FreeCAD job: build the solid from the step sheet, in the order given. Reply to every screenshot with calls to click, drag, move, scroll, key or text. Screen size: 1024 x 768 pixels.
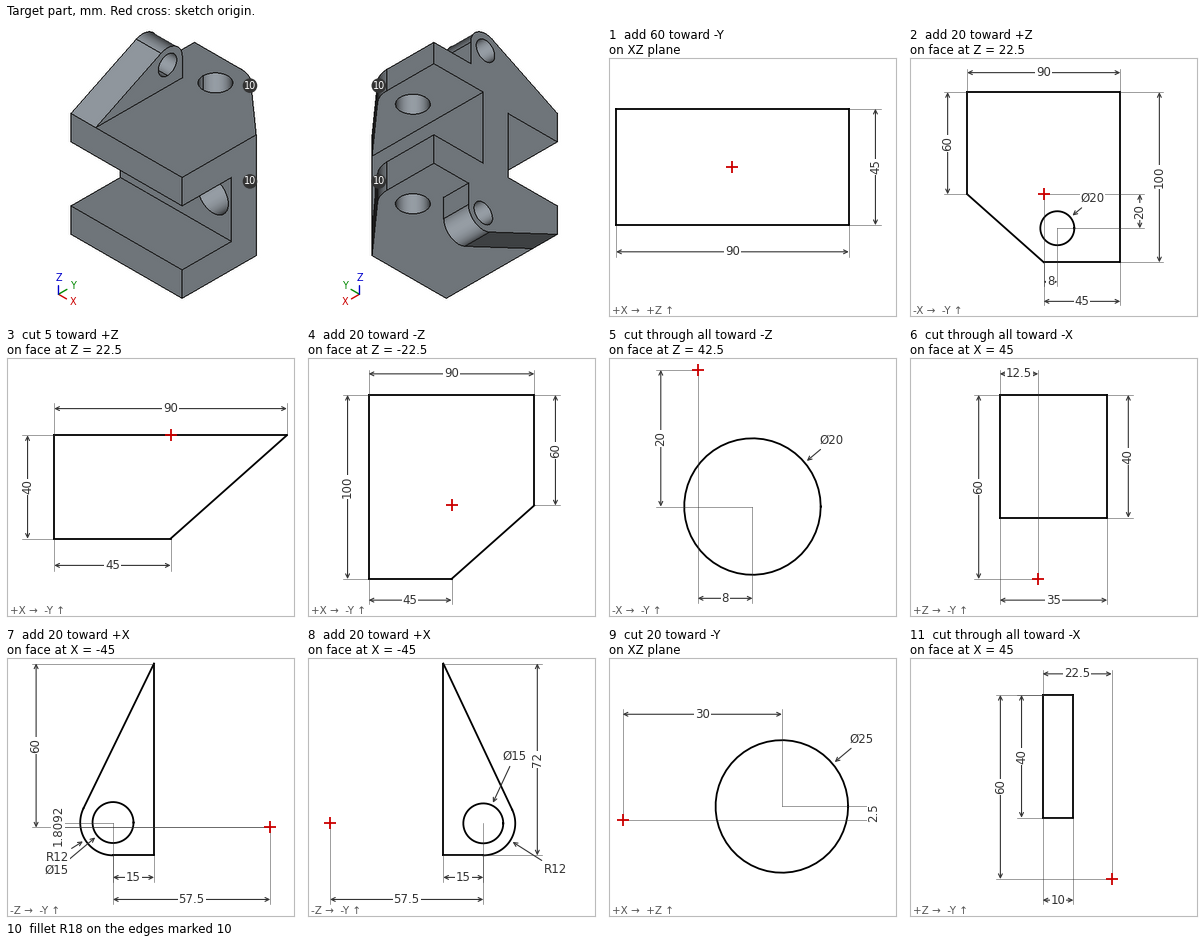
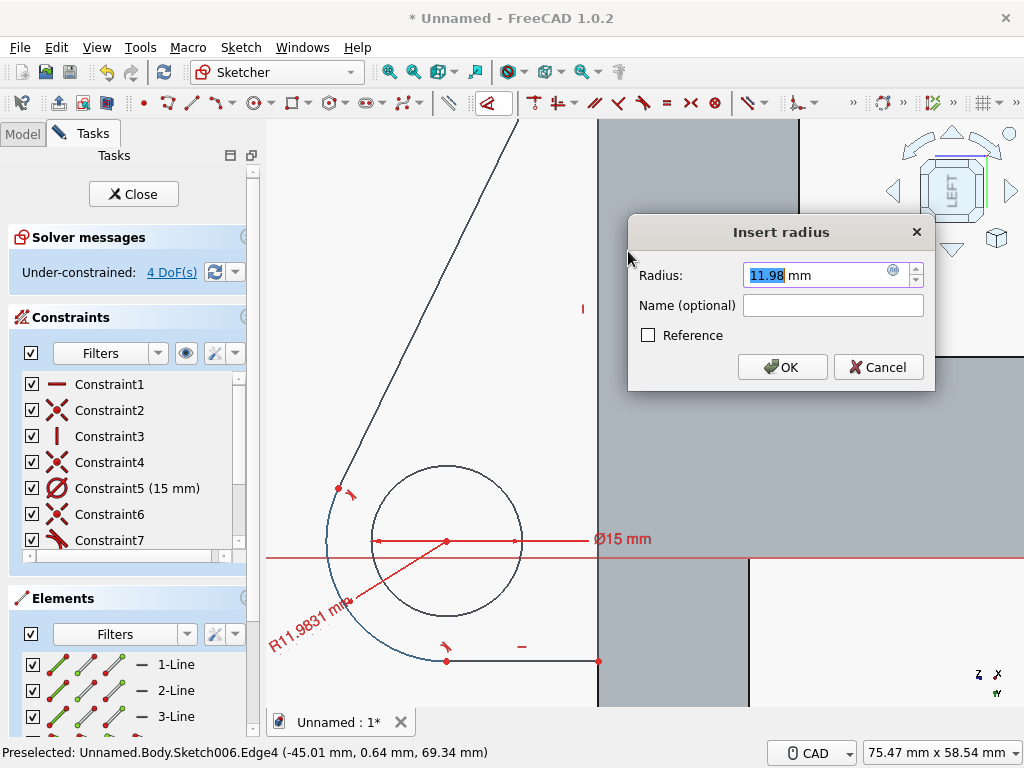
text(12)
key(Return)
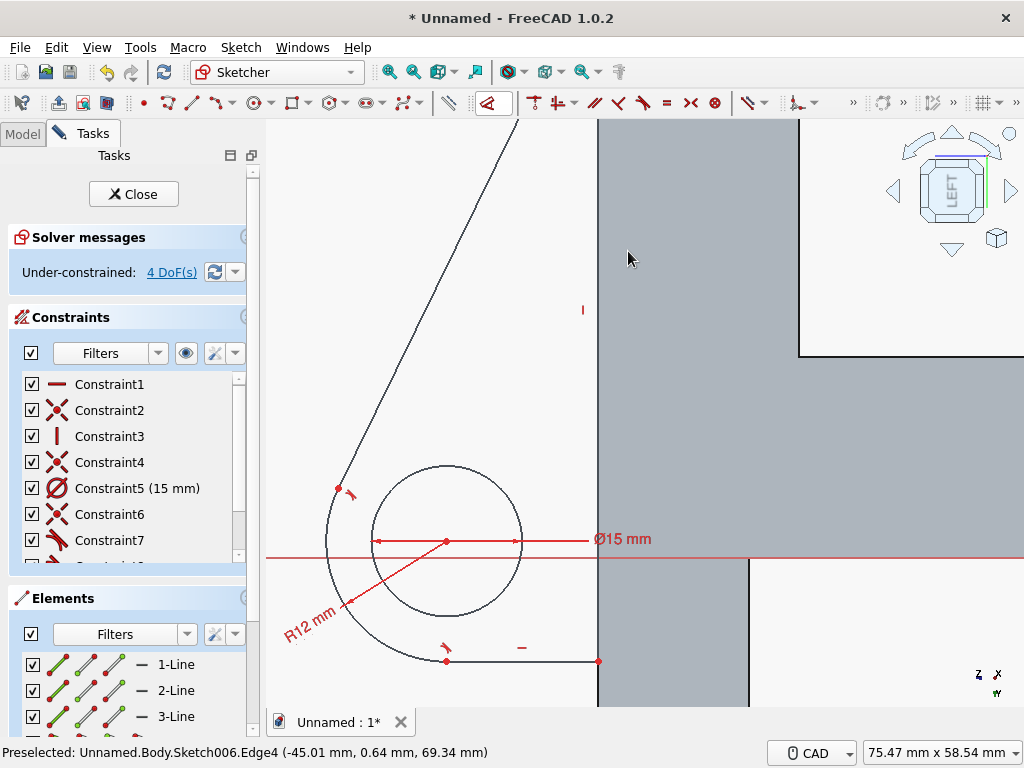
click(492, 662)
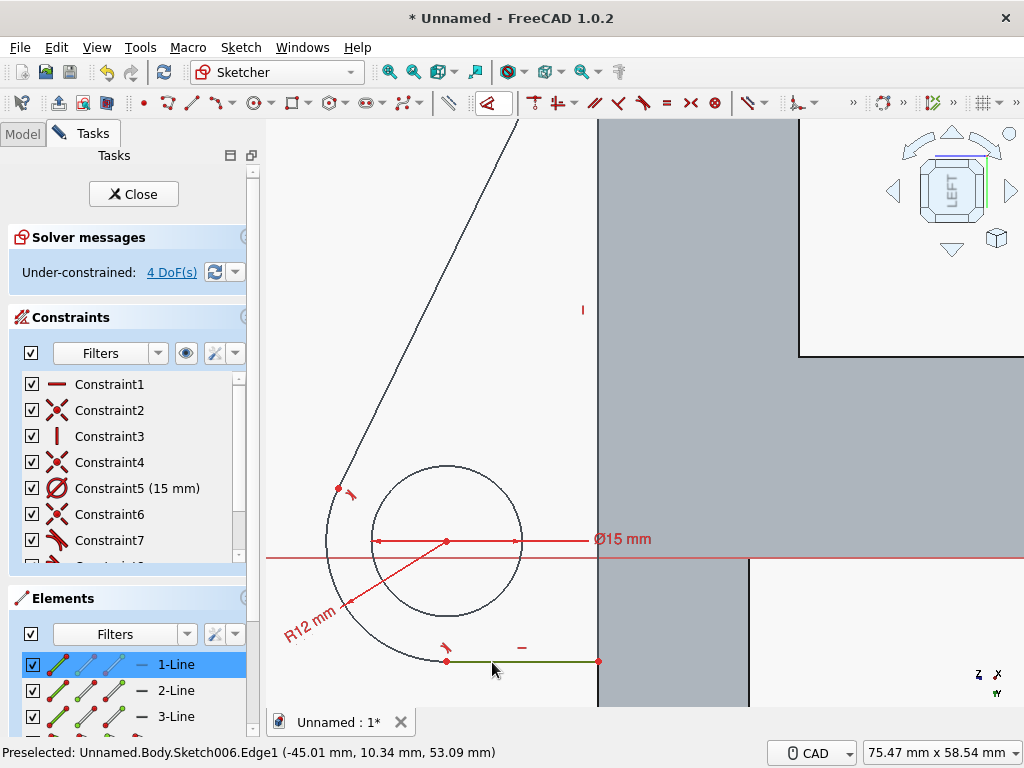
key(l)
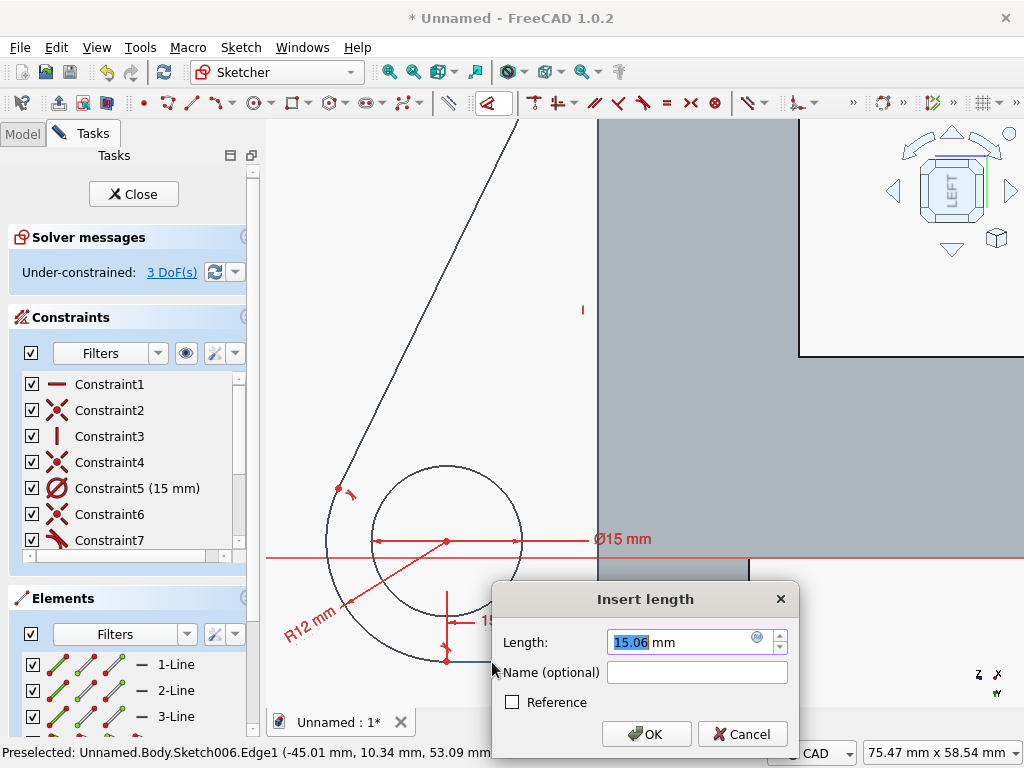
text(15)
key(Return)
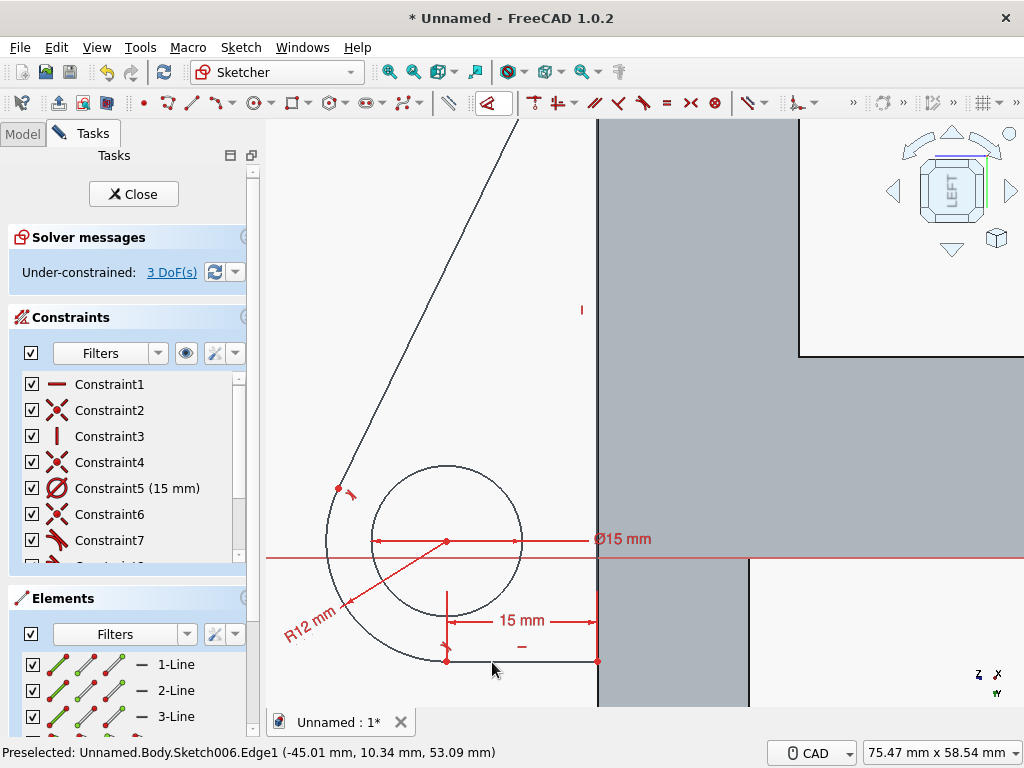
scroll(448, 541, down, 3)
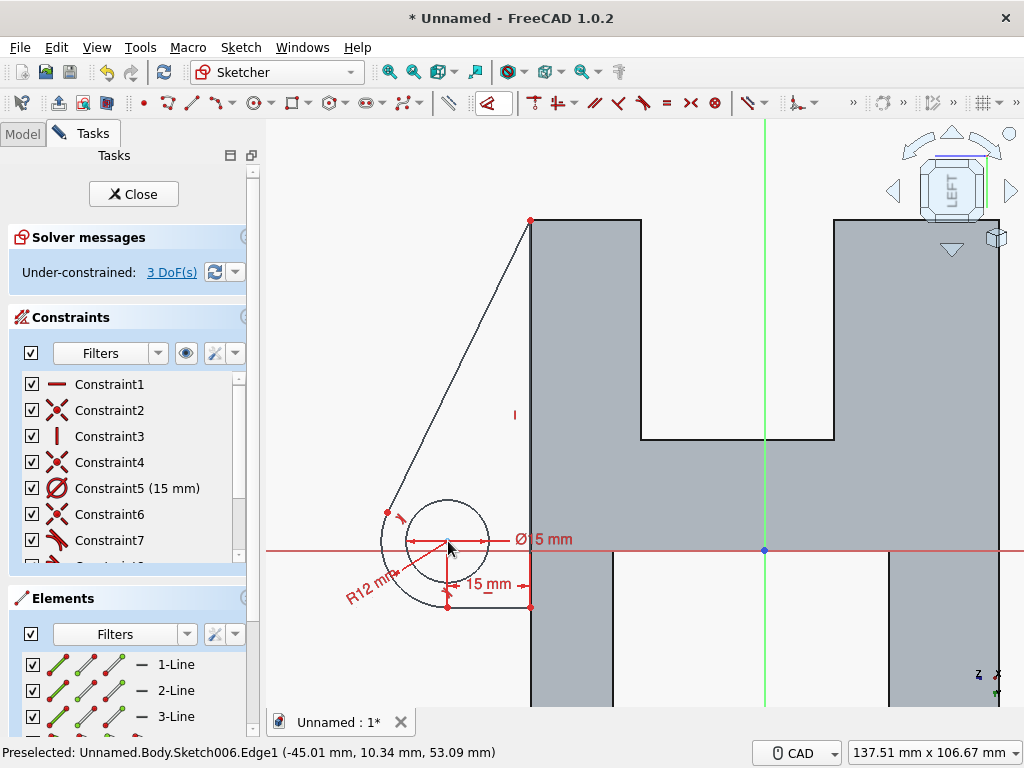
click(530, 220)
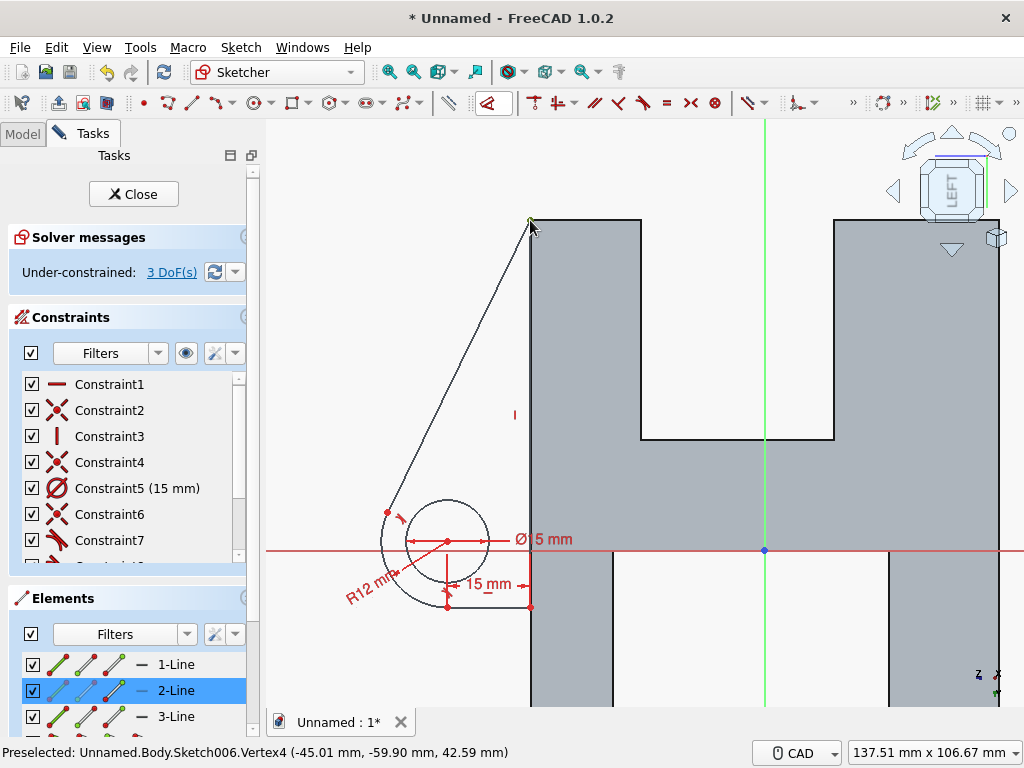
click(506, 104)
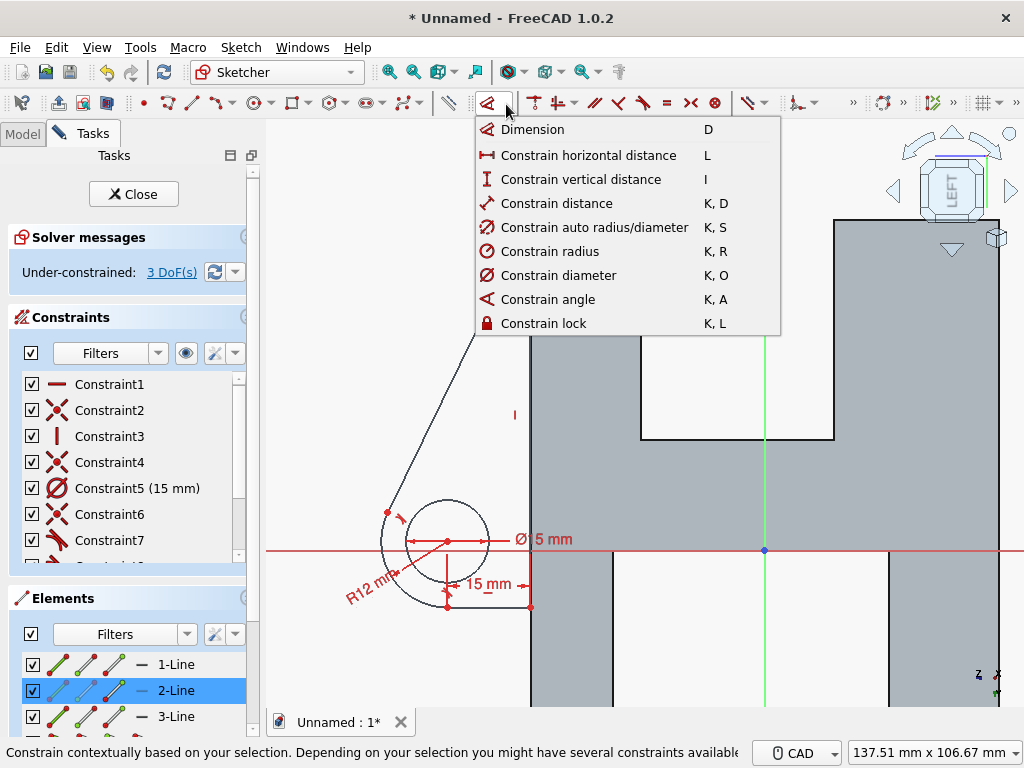
click(628, 179)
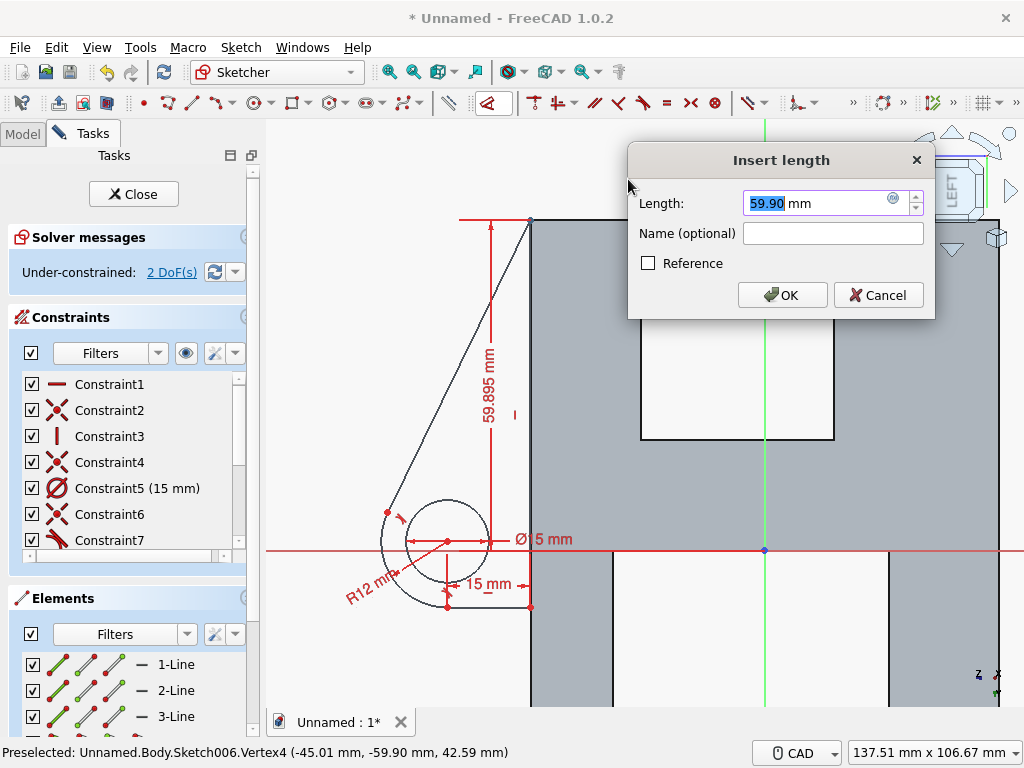
text(60)
key(Return)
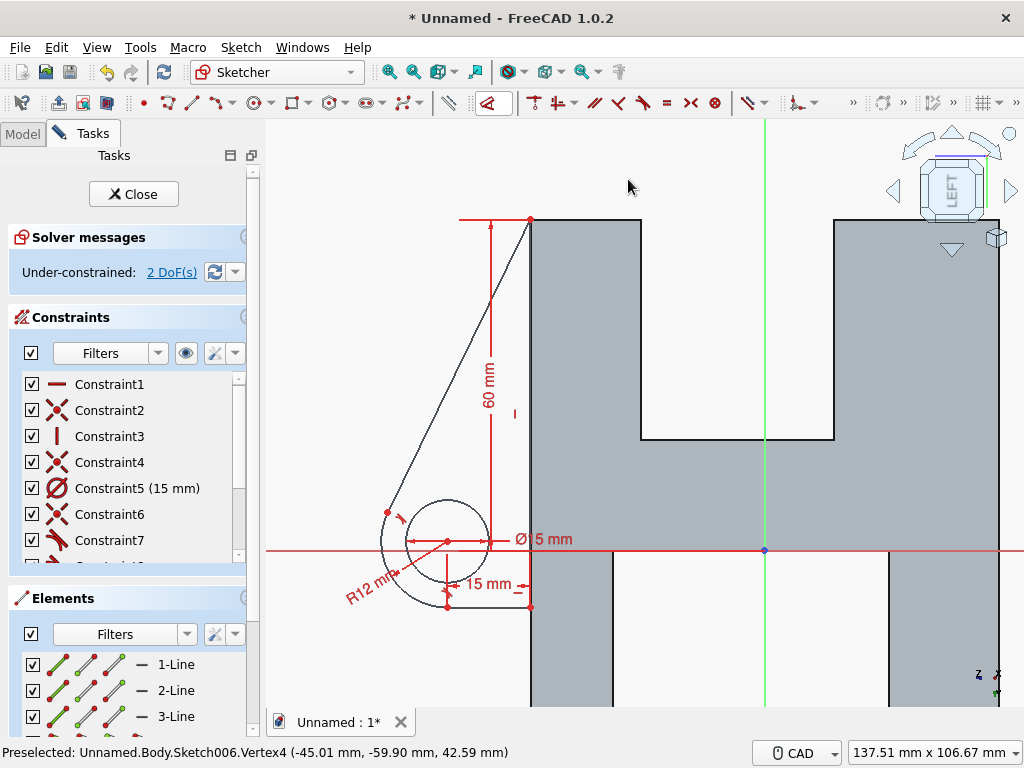
click(447, 541)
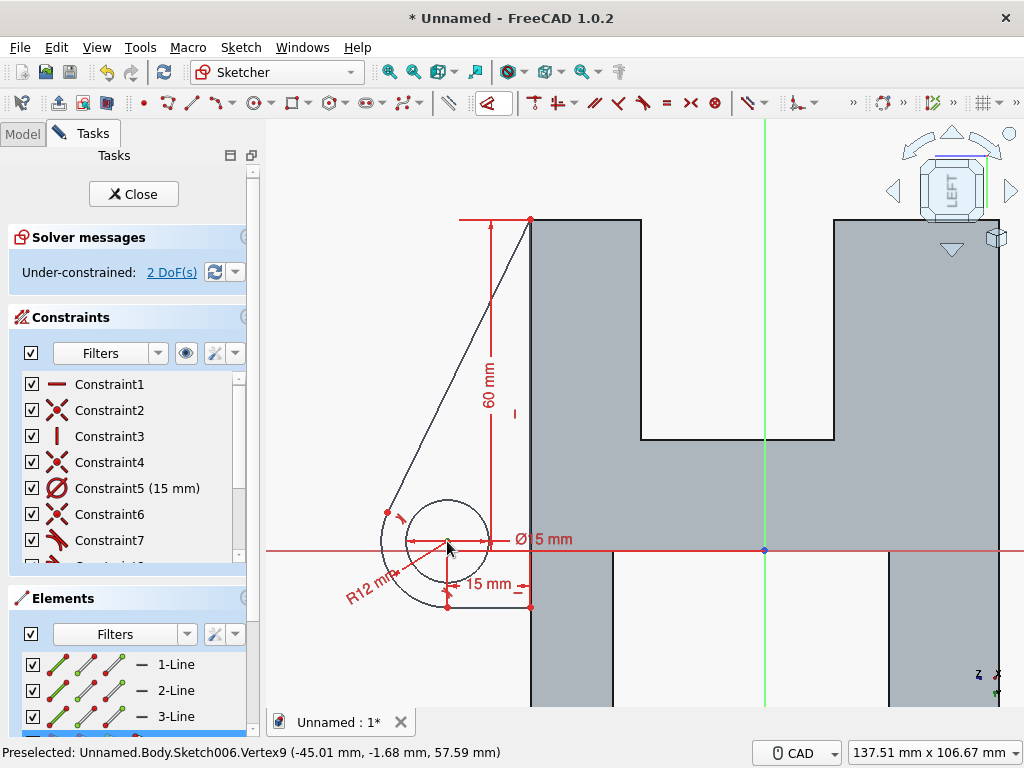
key(l)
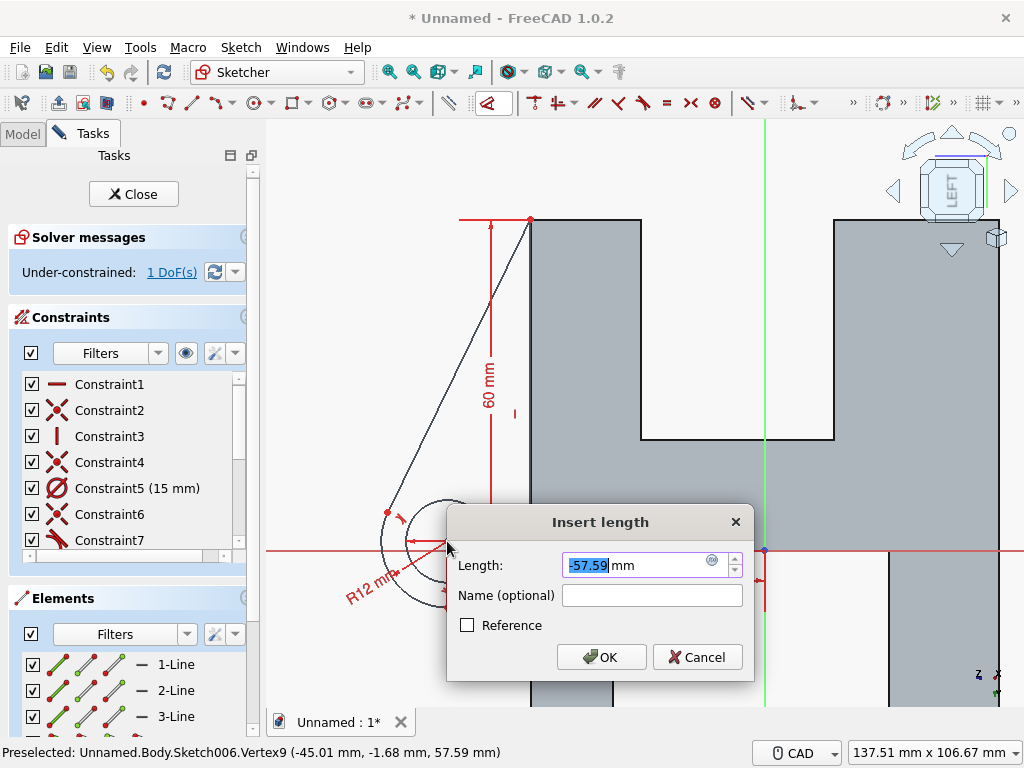
text(-57.5)
key(Return)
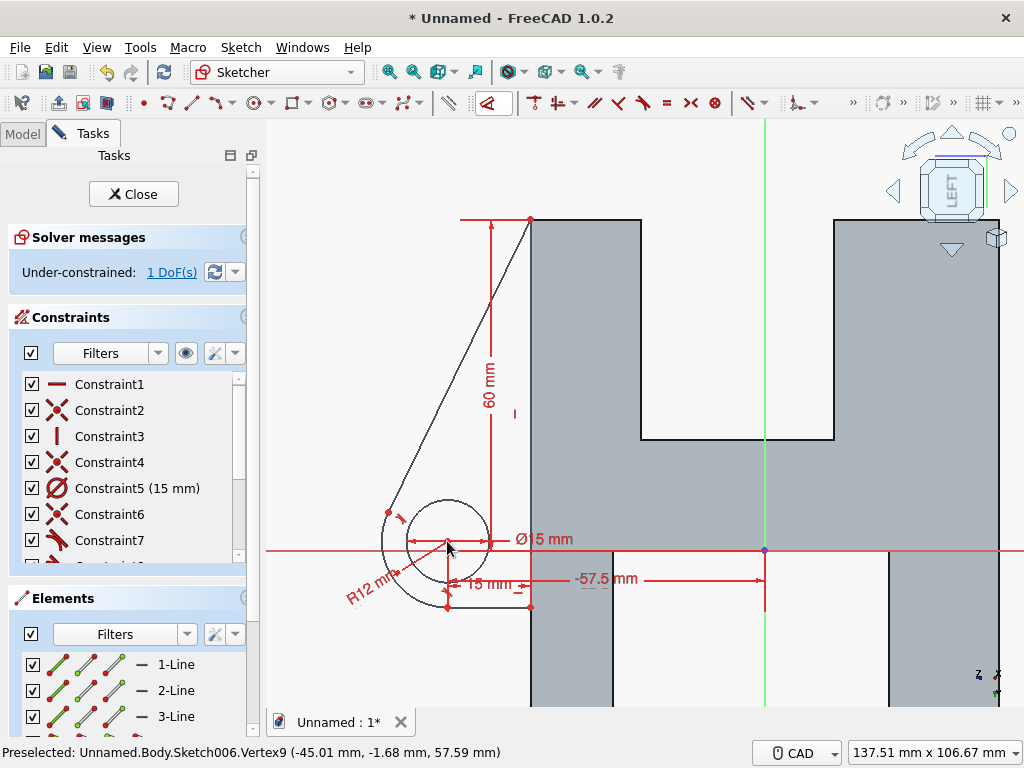
scroll(448, 541, up, 7)